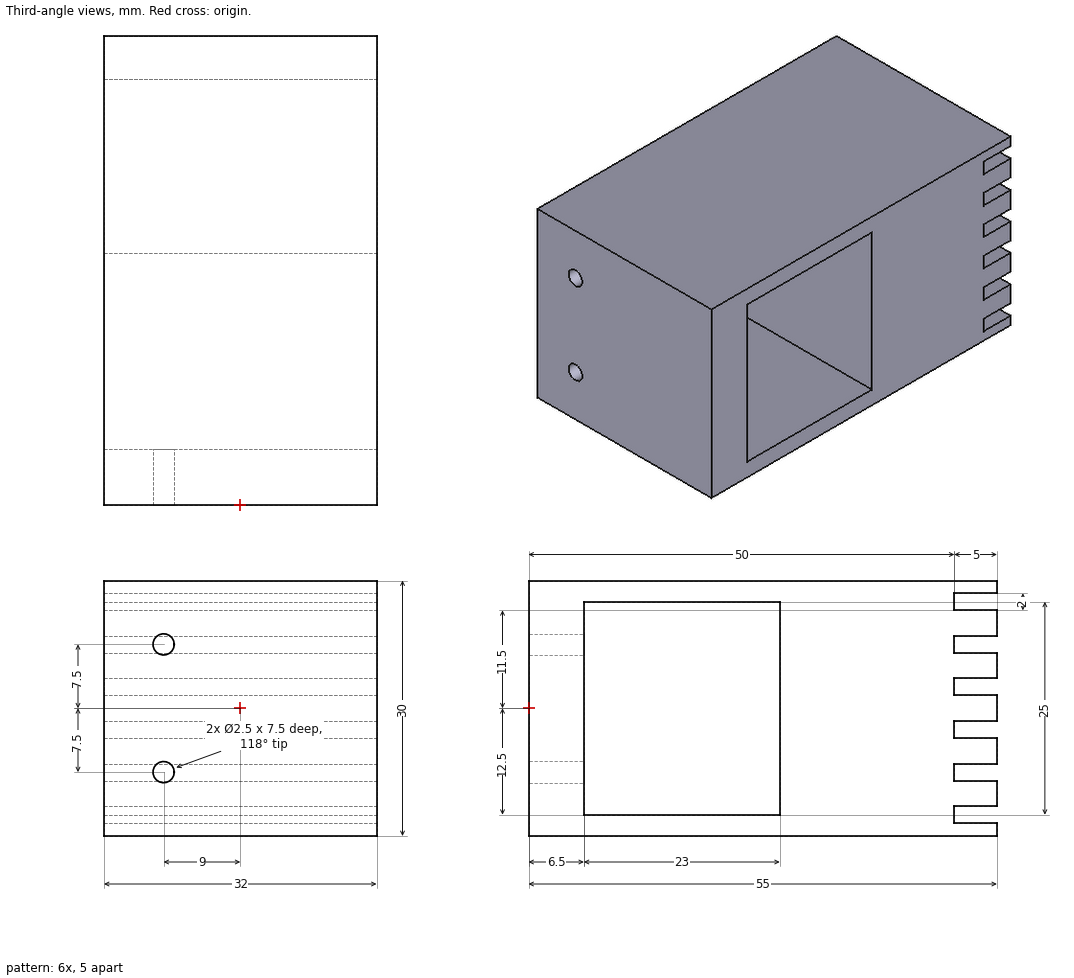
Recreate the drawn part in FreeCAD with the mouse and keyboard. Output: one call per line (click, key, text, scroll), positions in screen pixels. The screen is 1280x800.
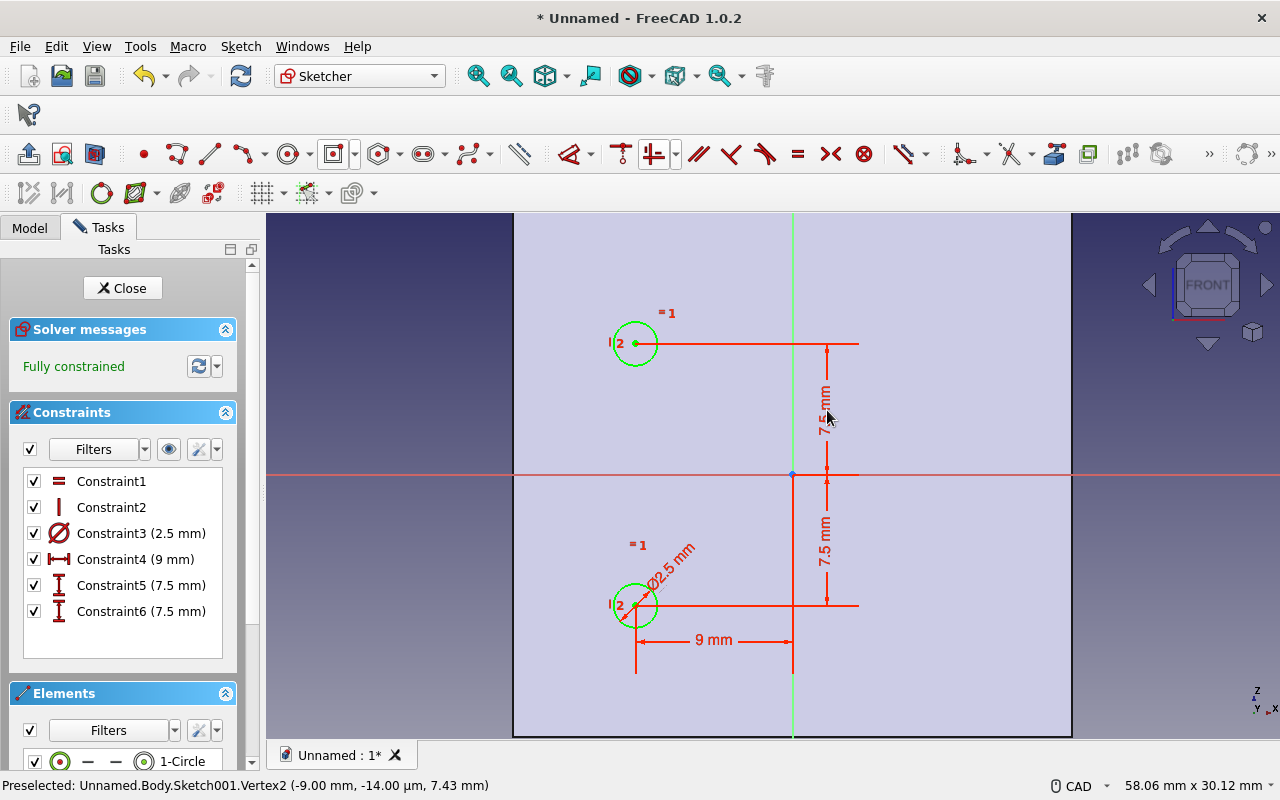
click(123, 288)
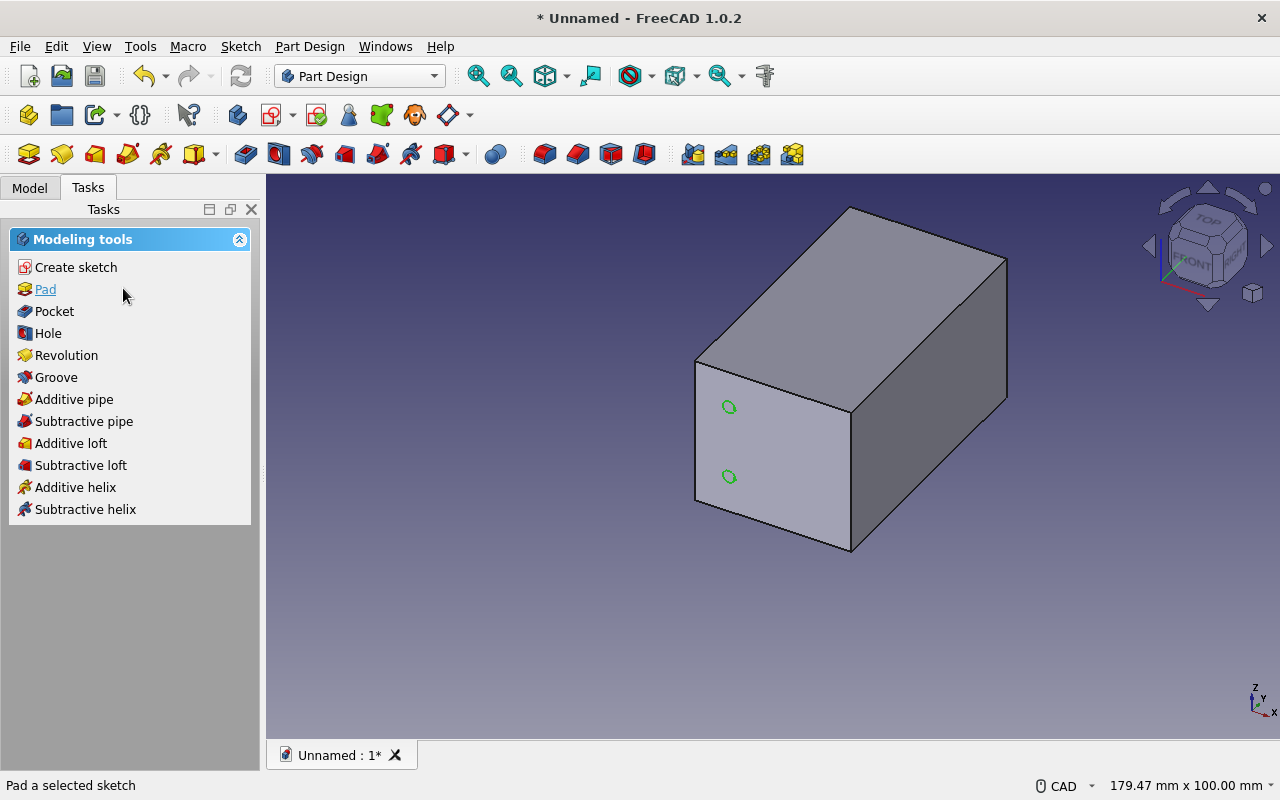
click(279, 154)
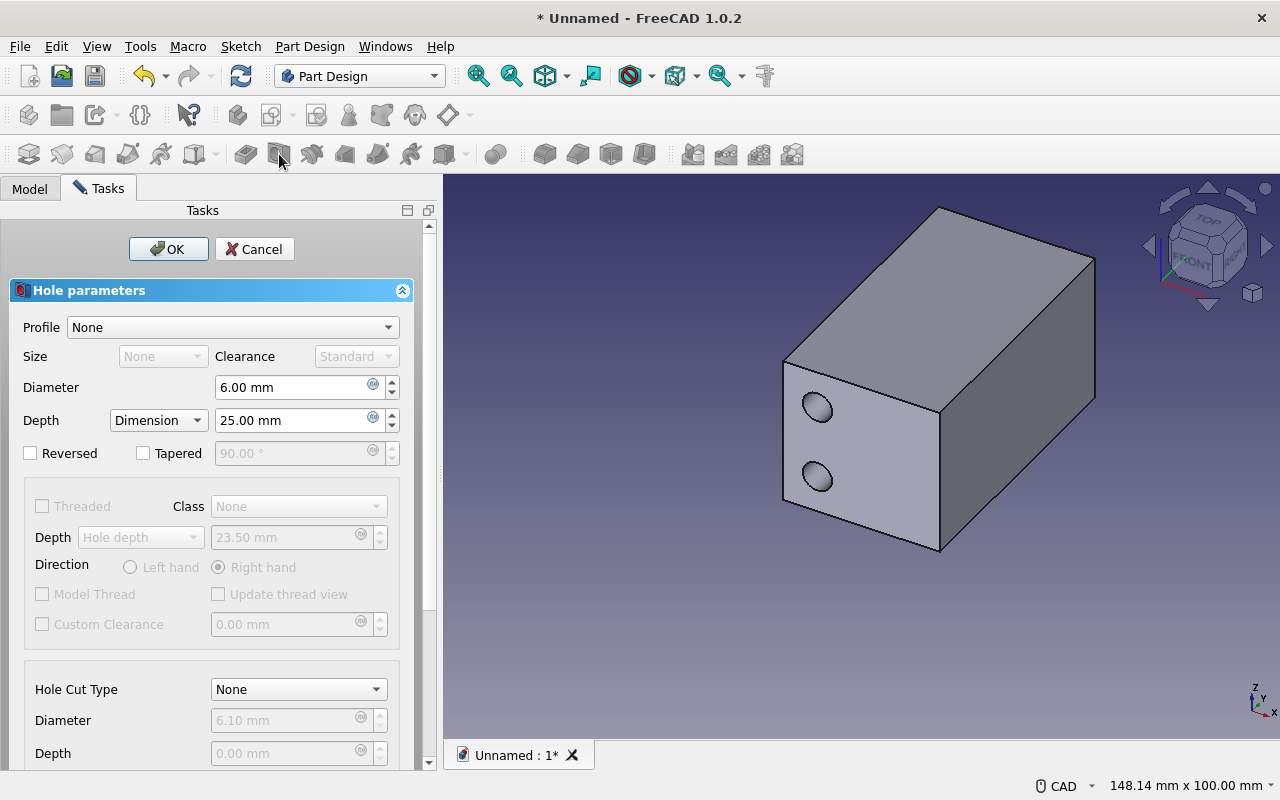
triple_click(300, 388)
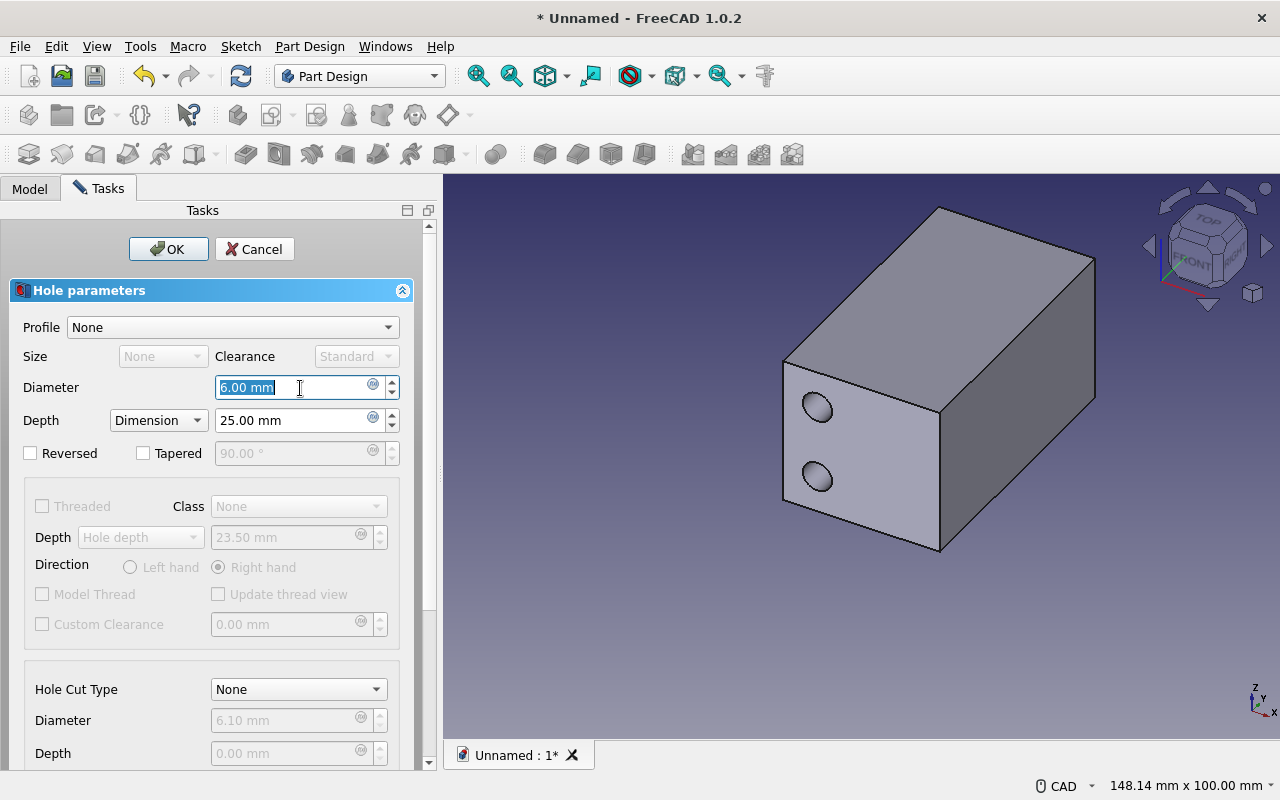
text(2.5)
key(Tab)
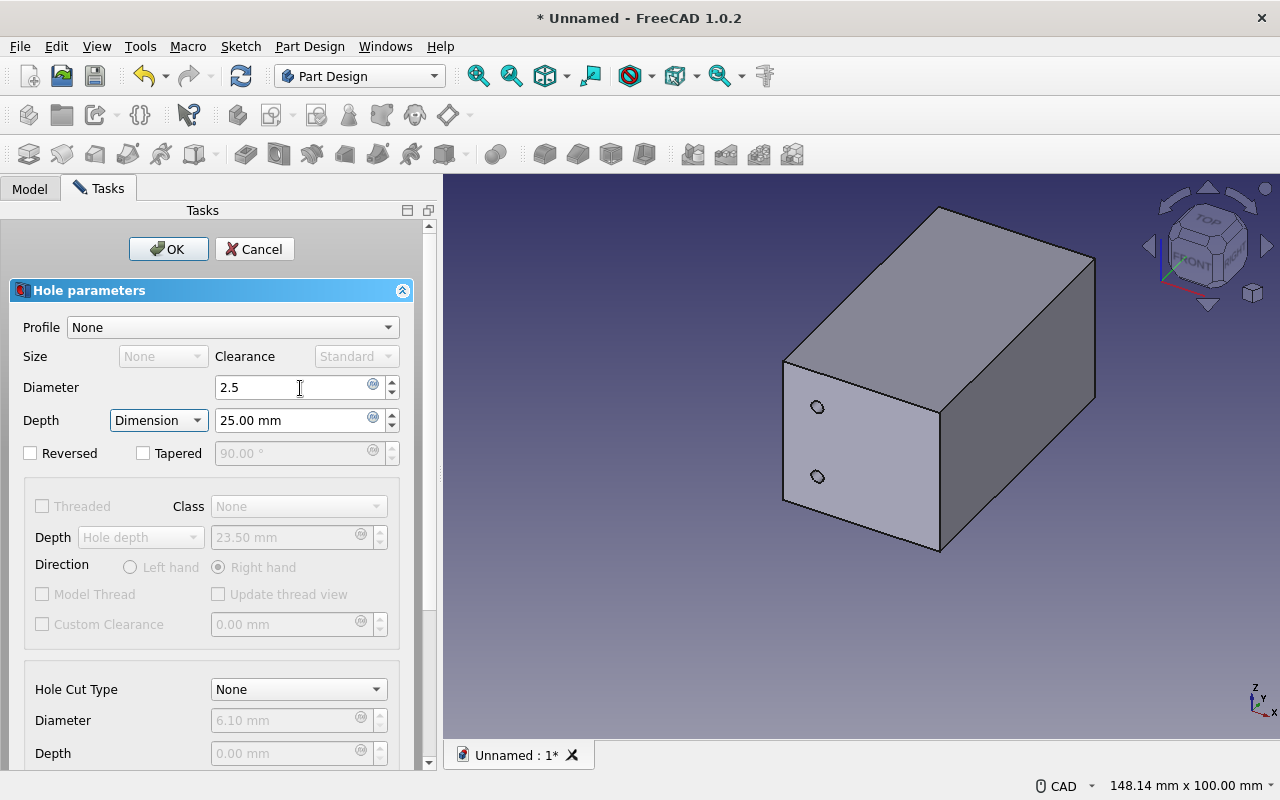
triple_click(300, 420)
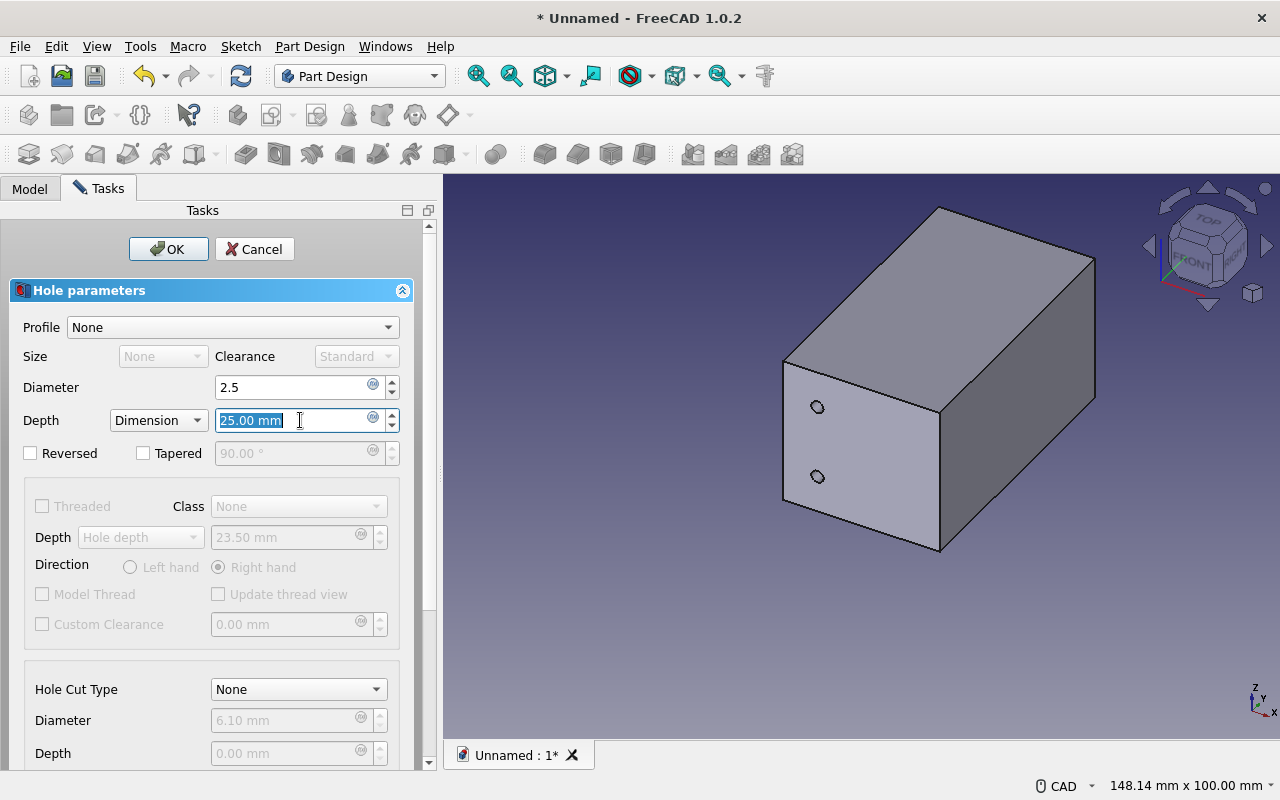
text(7.5)
key(Tab)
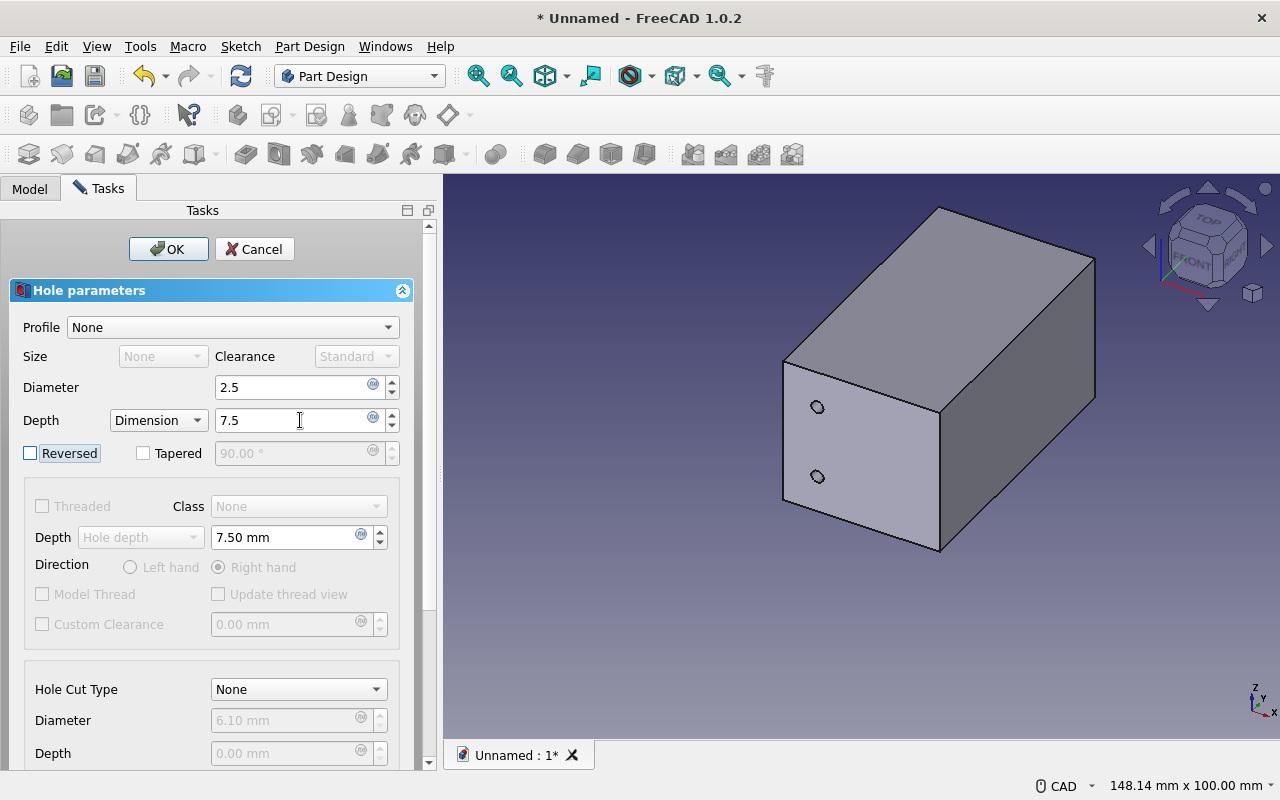
click(169, 249)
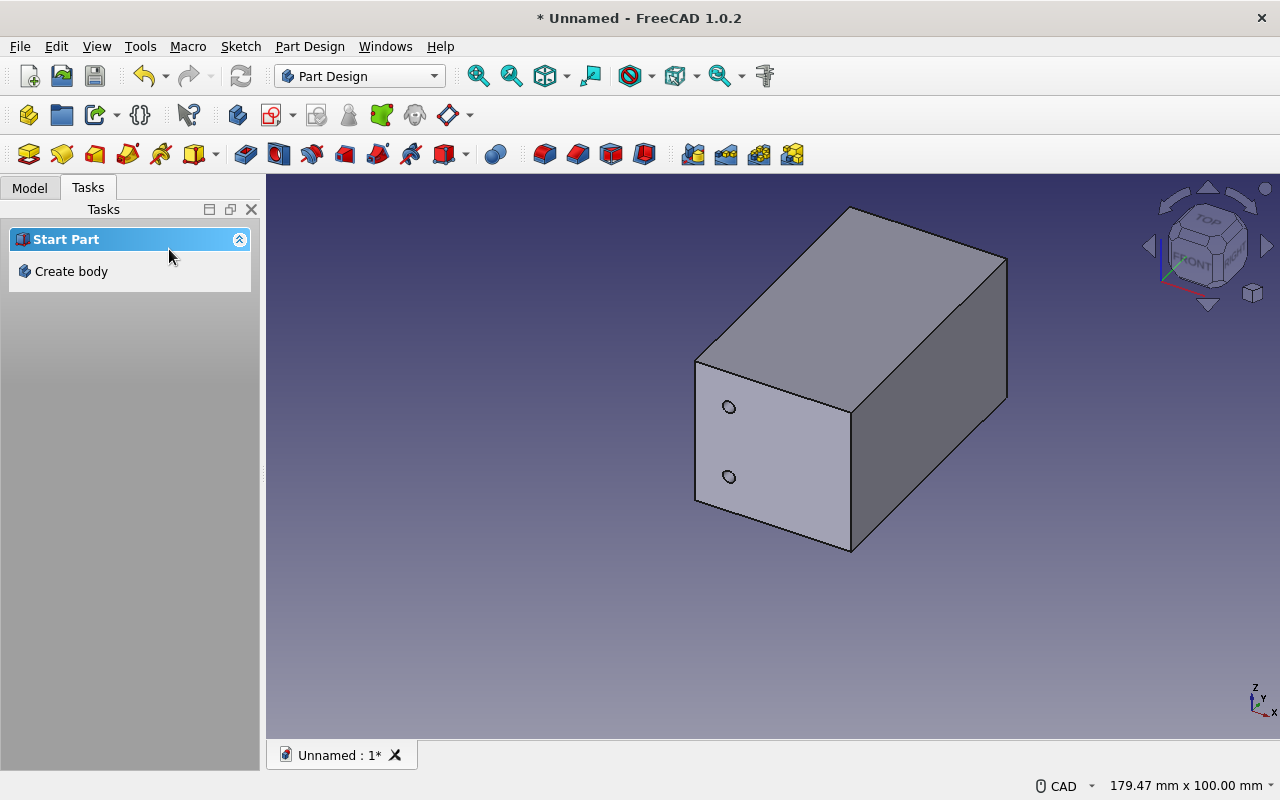
click(951, 382)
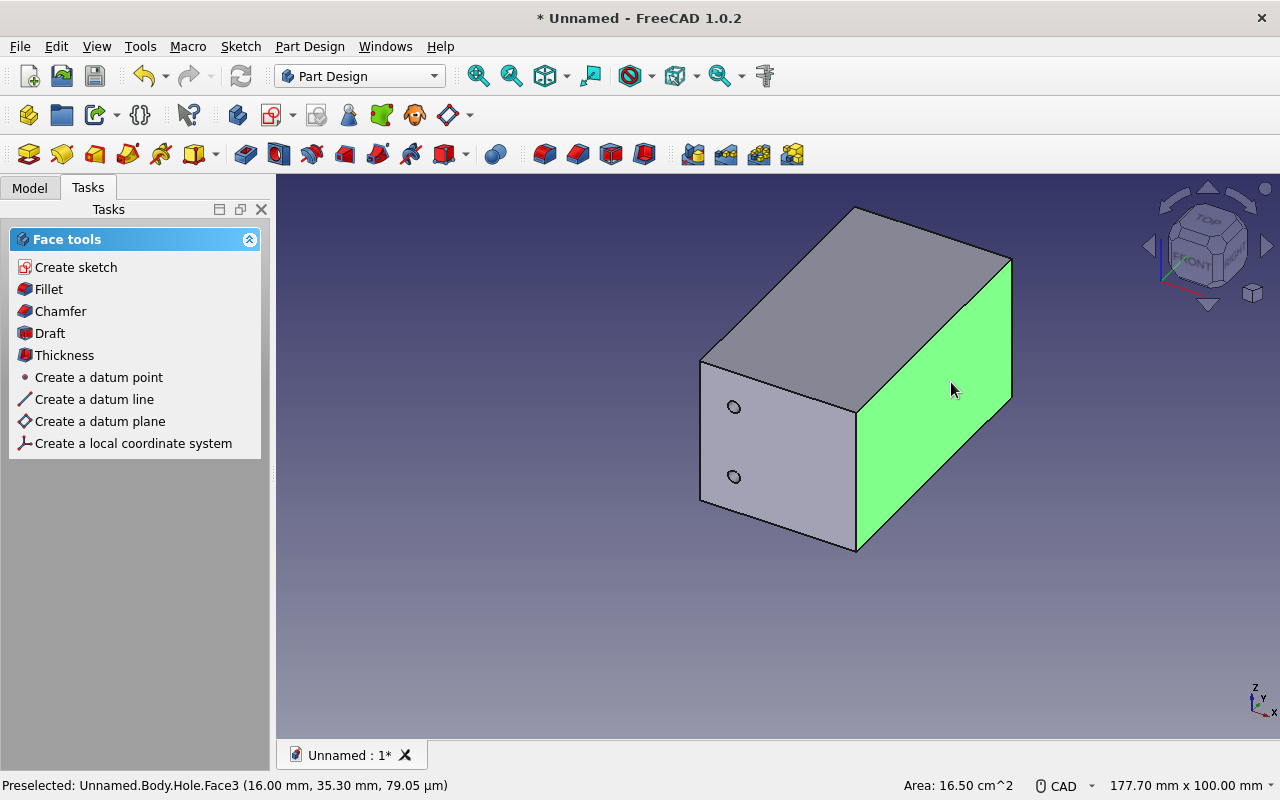
click(270, 116)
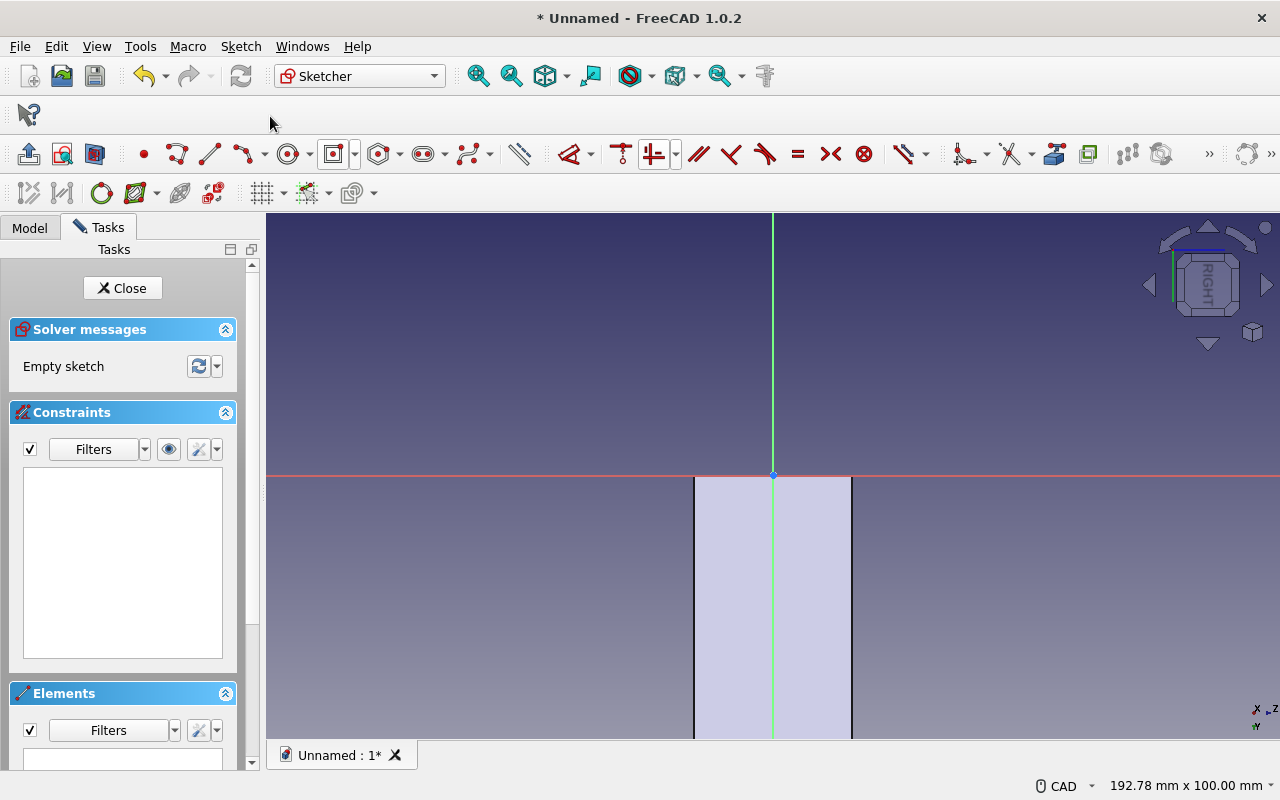
scroll(829, 617, up, 4)